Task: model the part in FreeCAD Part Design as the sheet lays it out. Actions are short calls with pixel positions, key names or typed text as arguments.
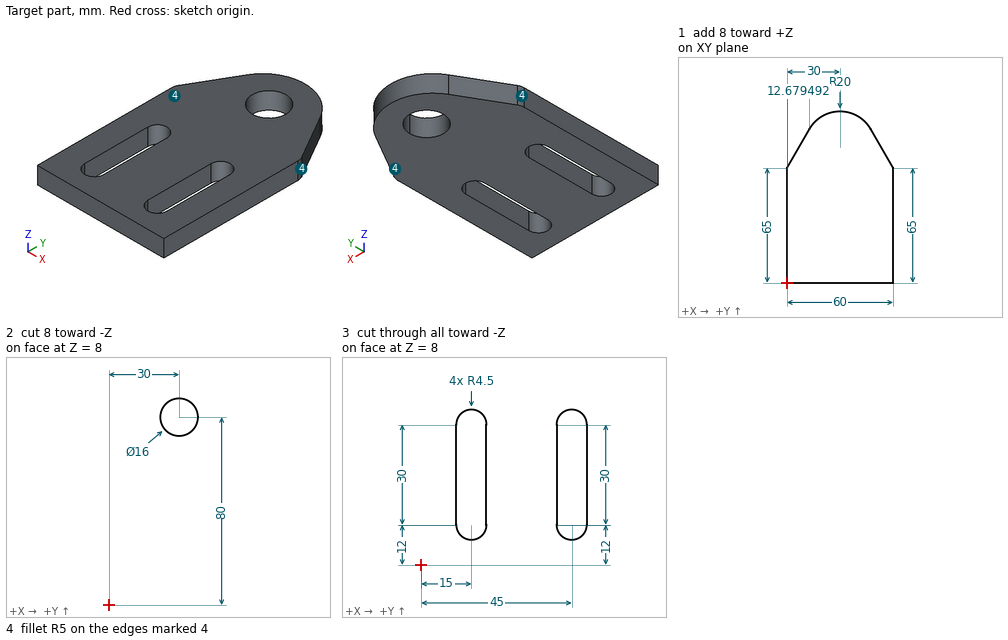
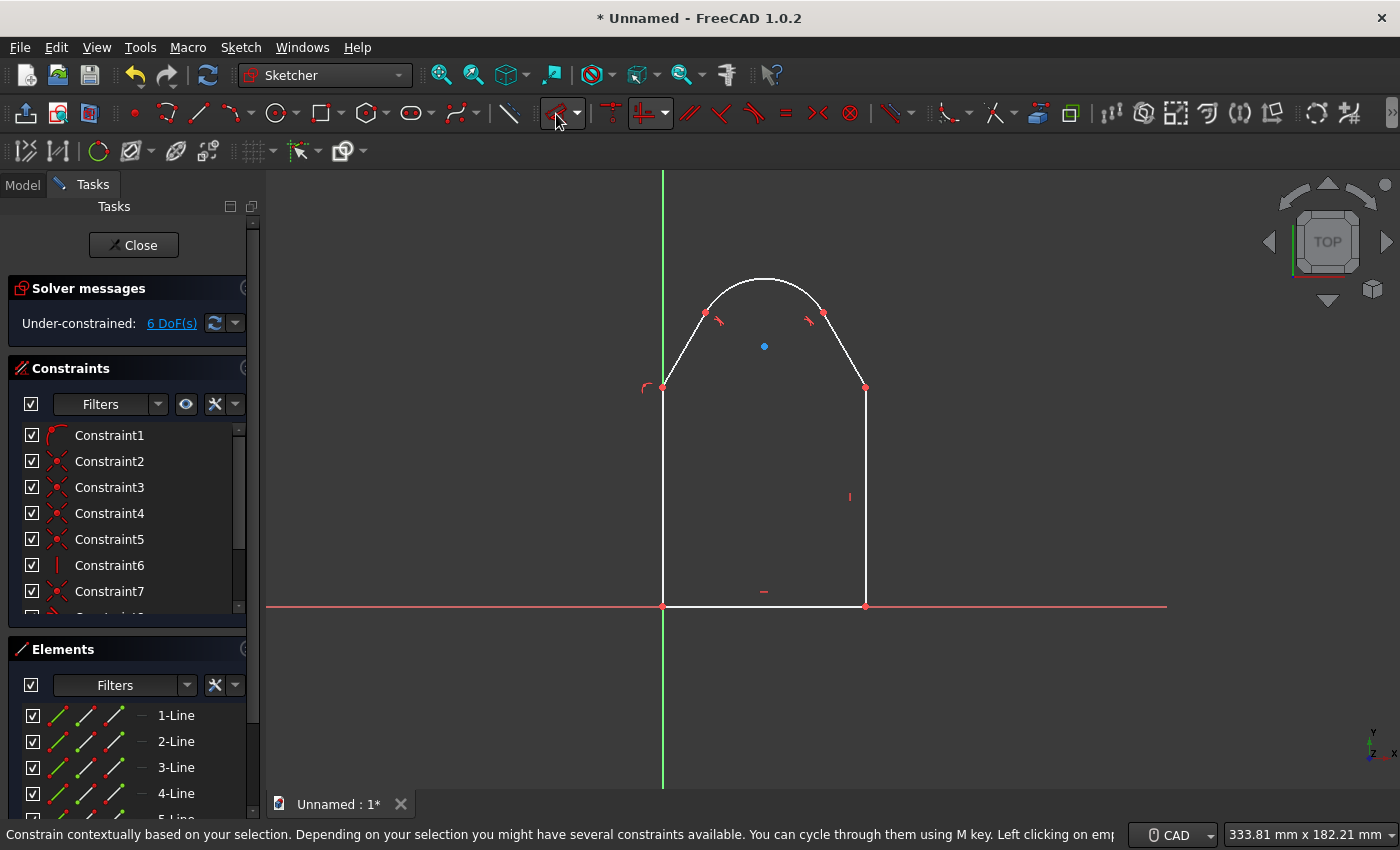
click(792, 285)
click(805, 256)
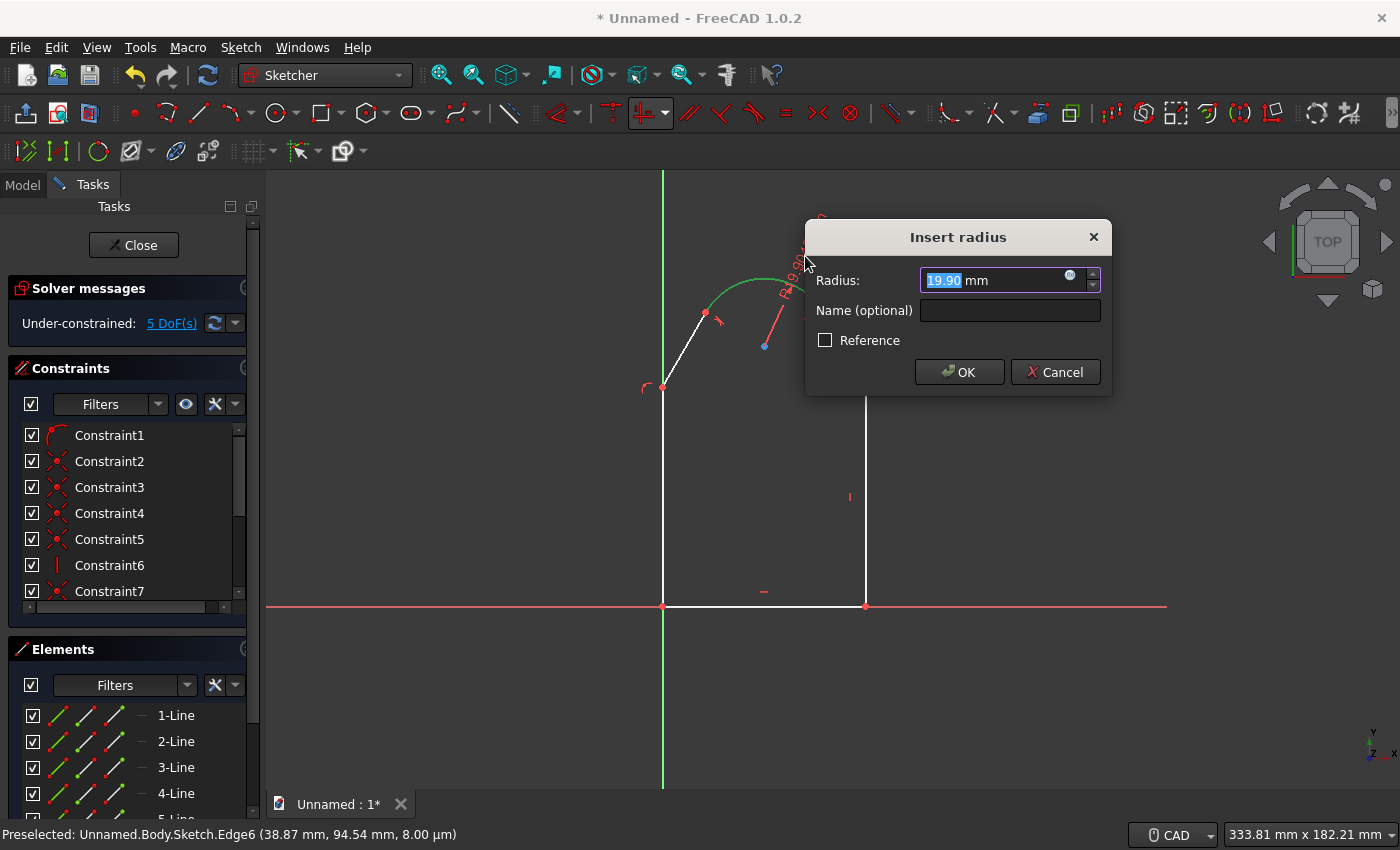
text(20)
key(Return)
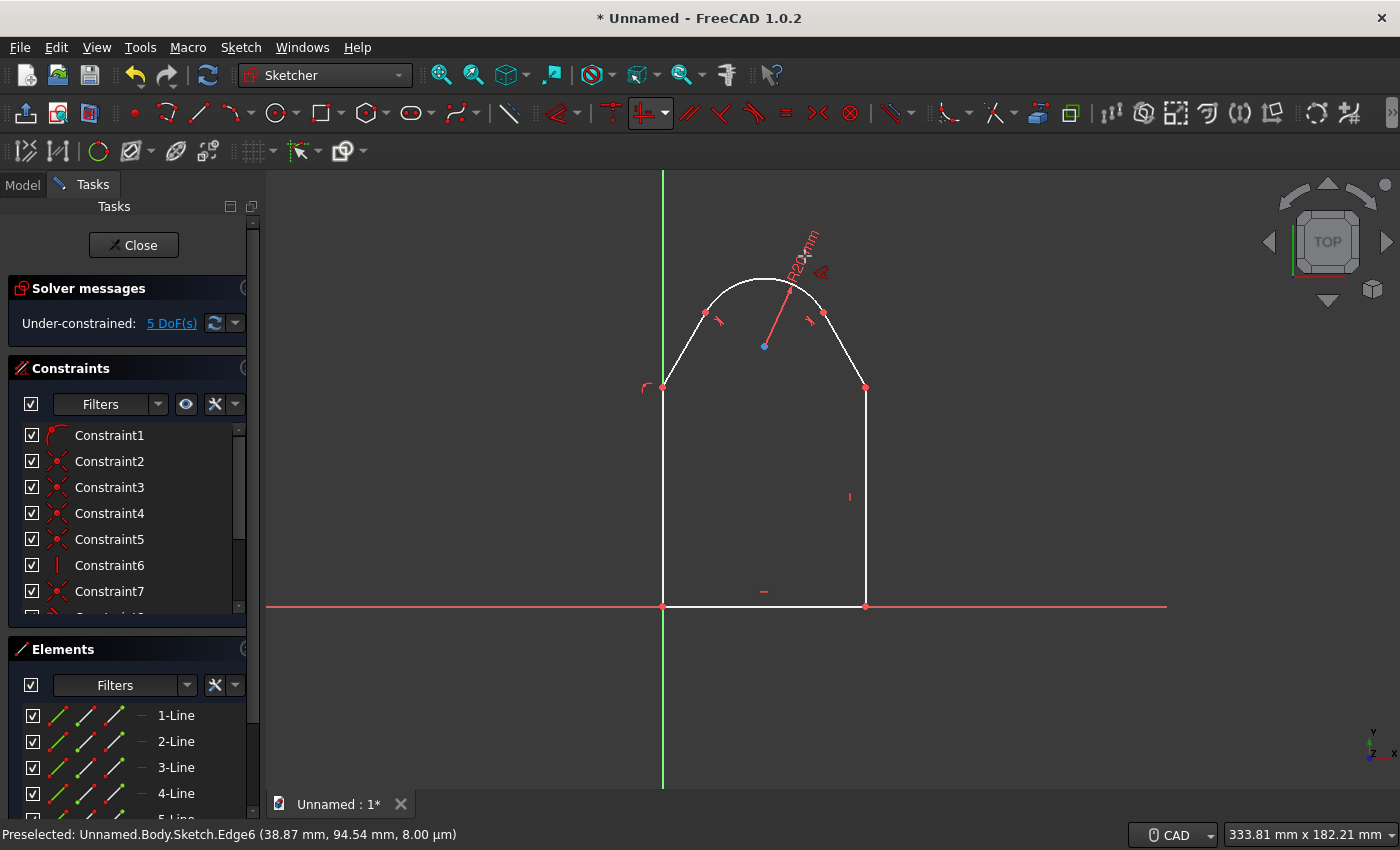
click(663, 453)
click(629, 497)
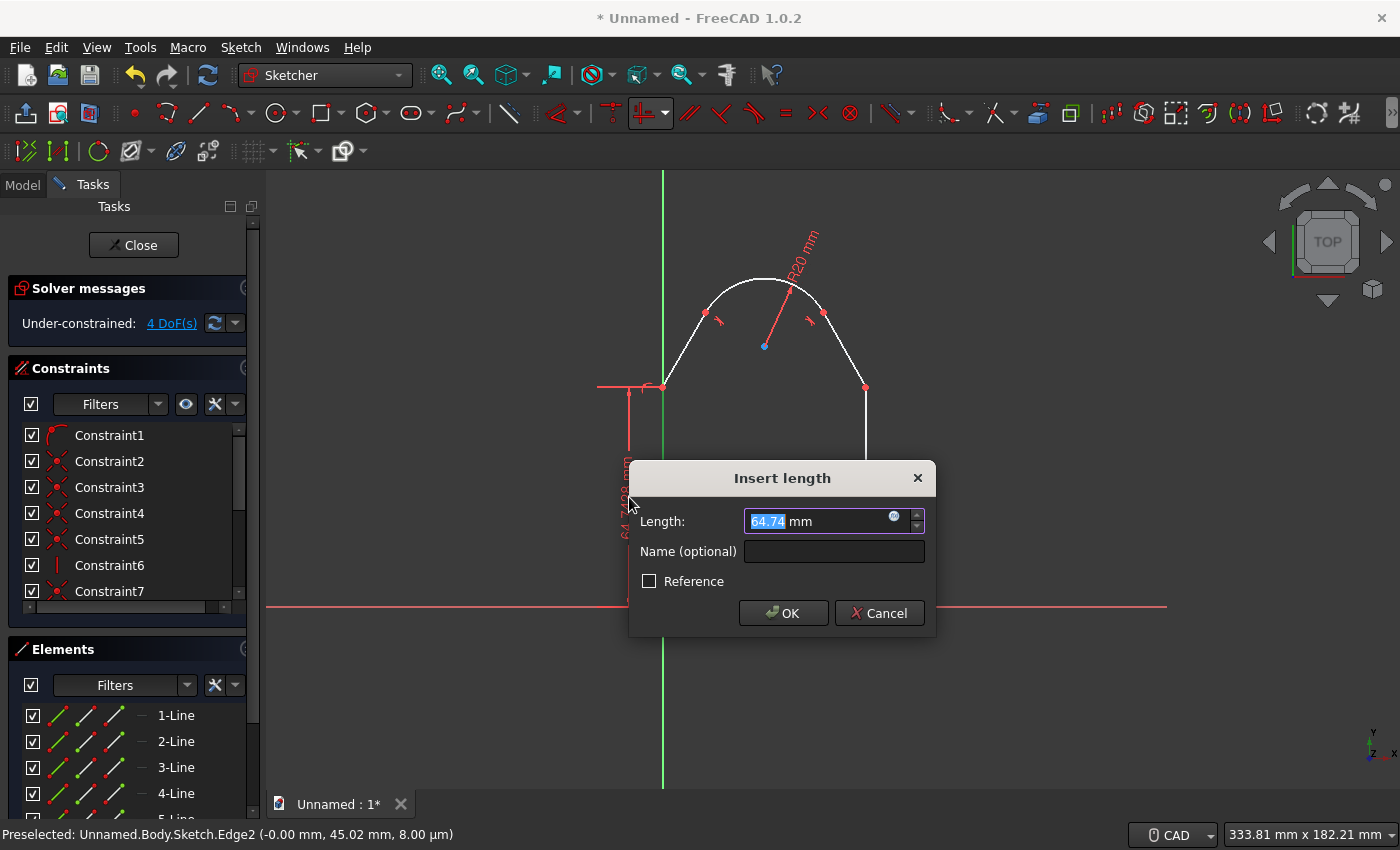
text(65)
key(Return)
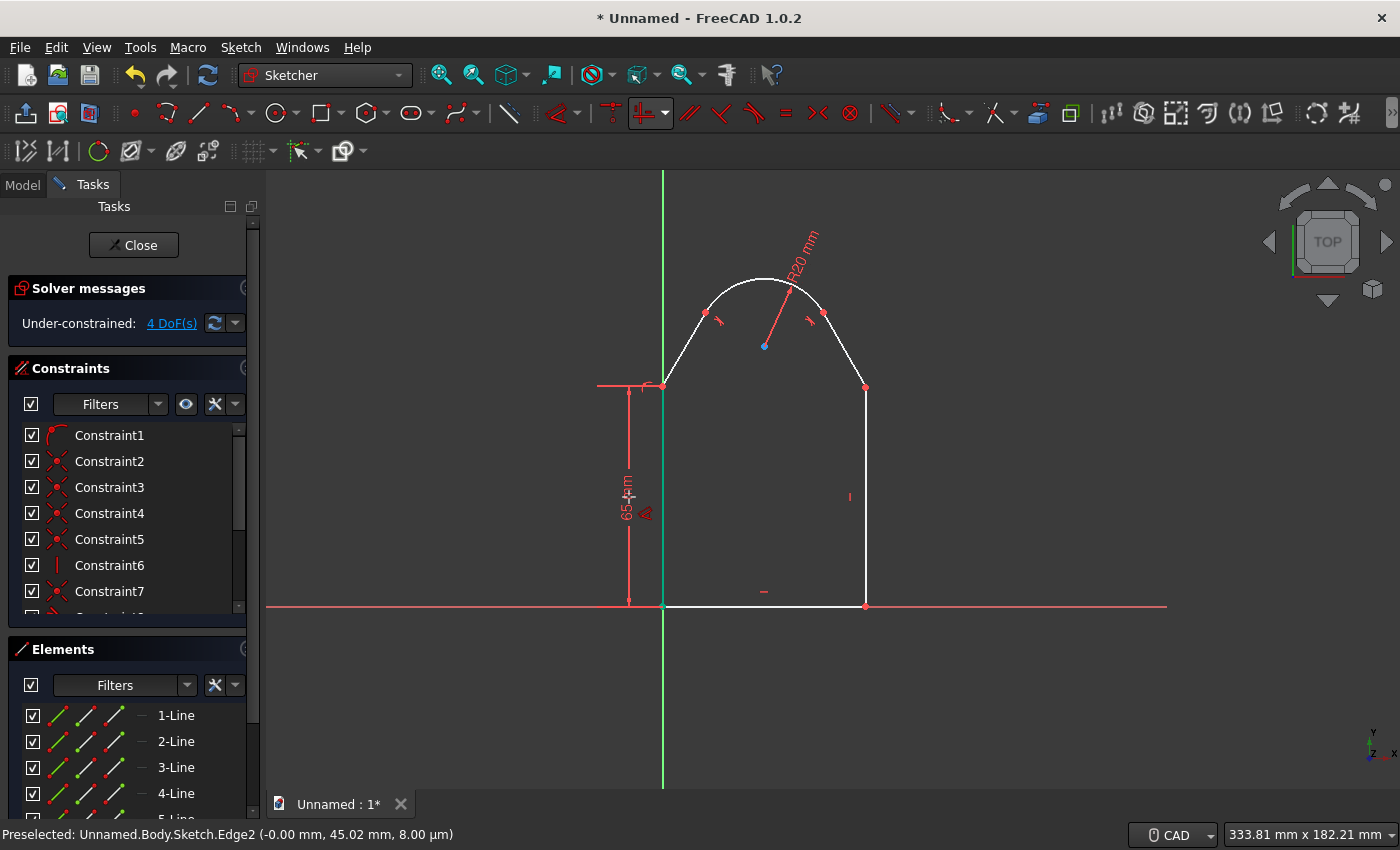
click(724, 607)
click(764, 641)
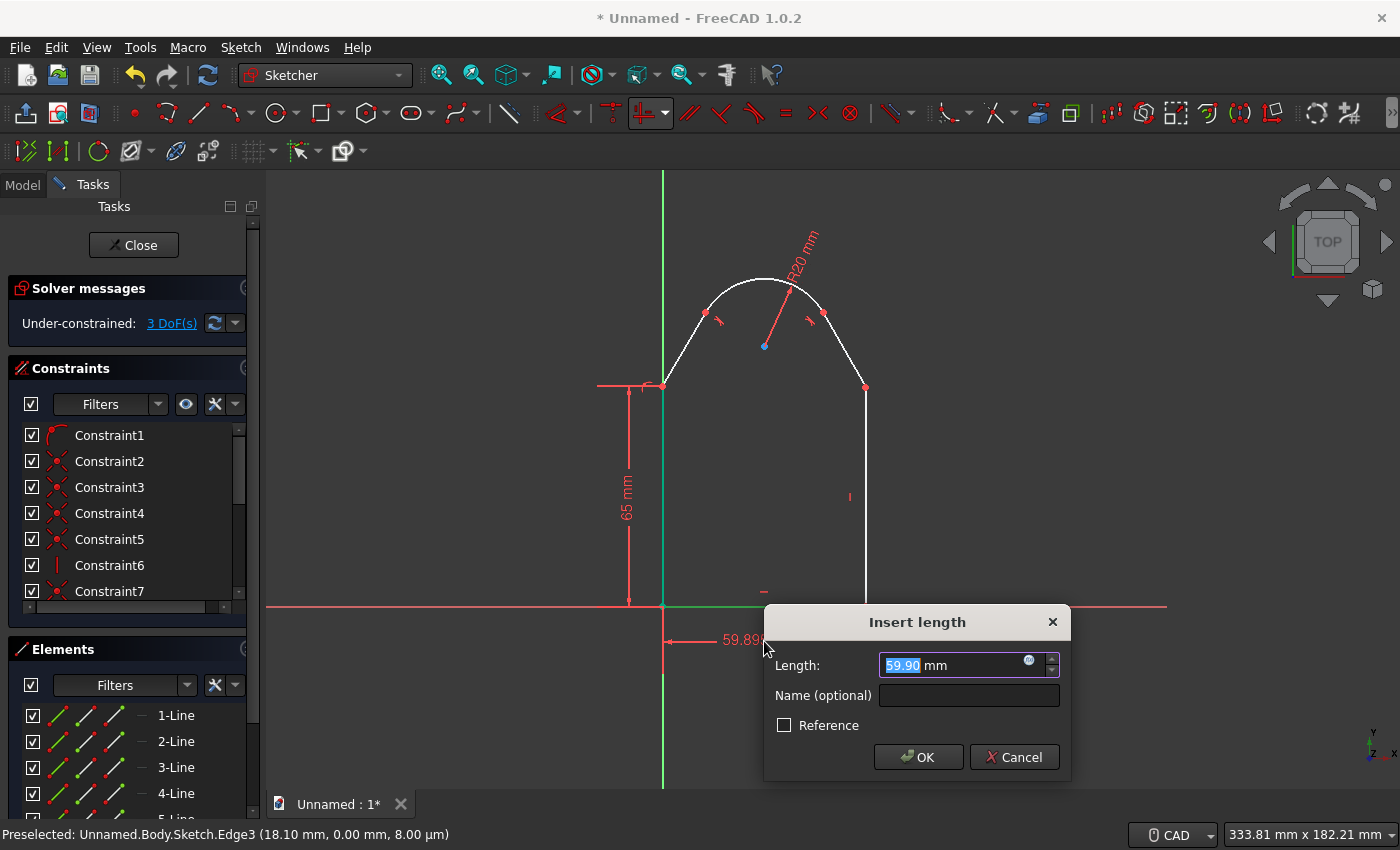
text(60)
key(Return)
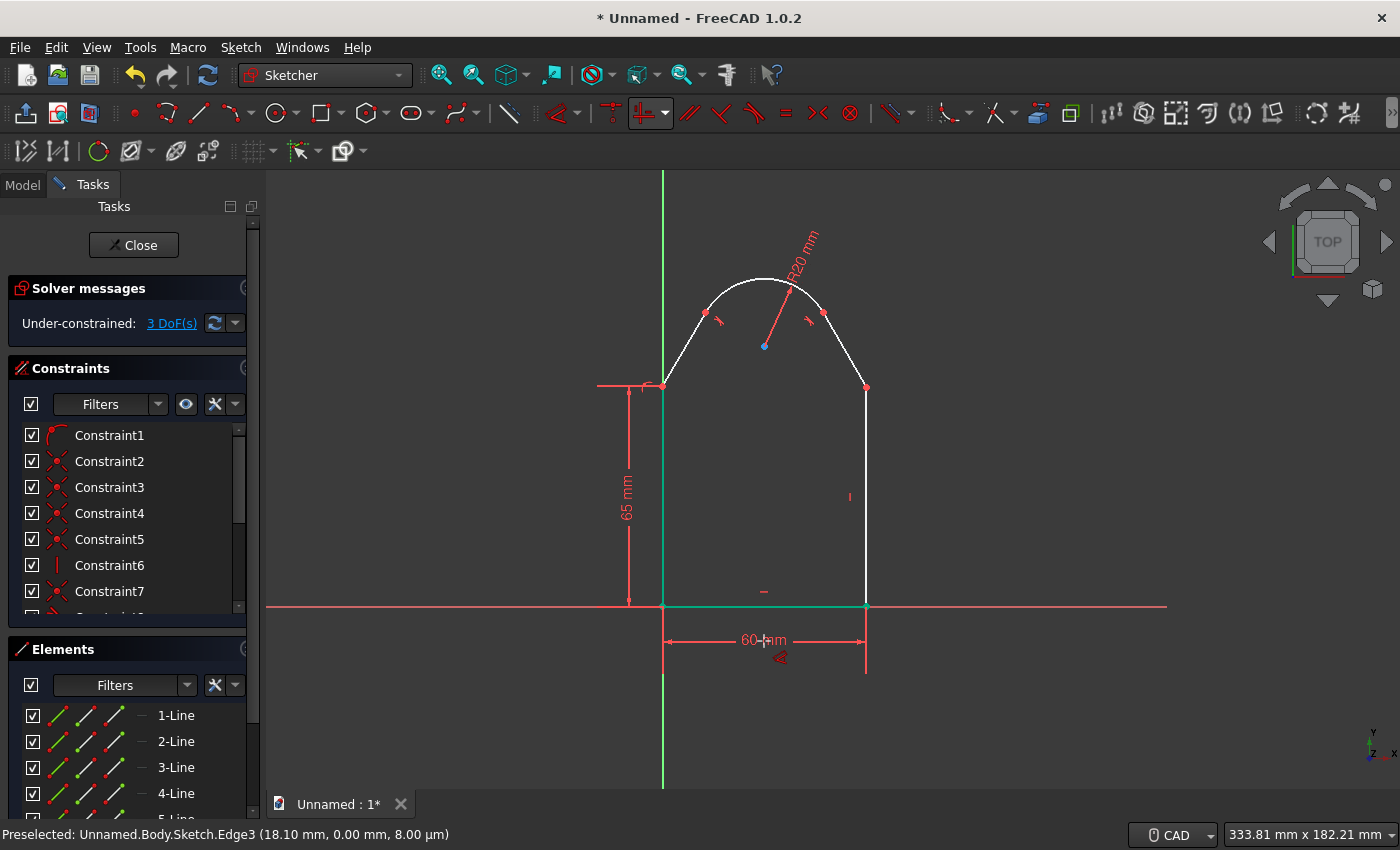
click(866, 541)
click(900, 497)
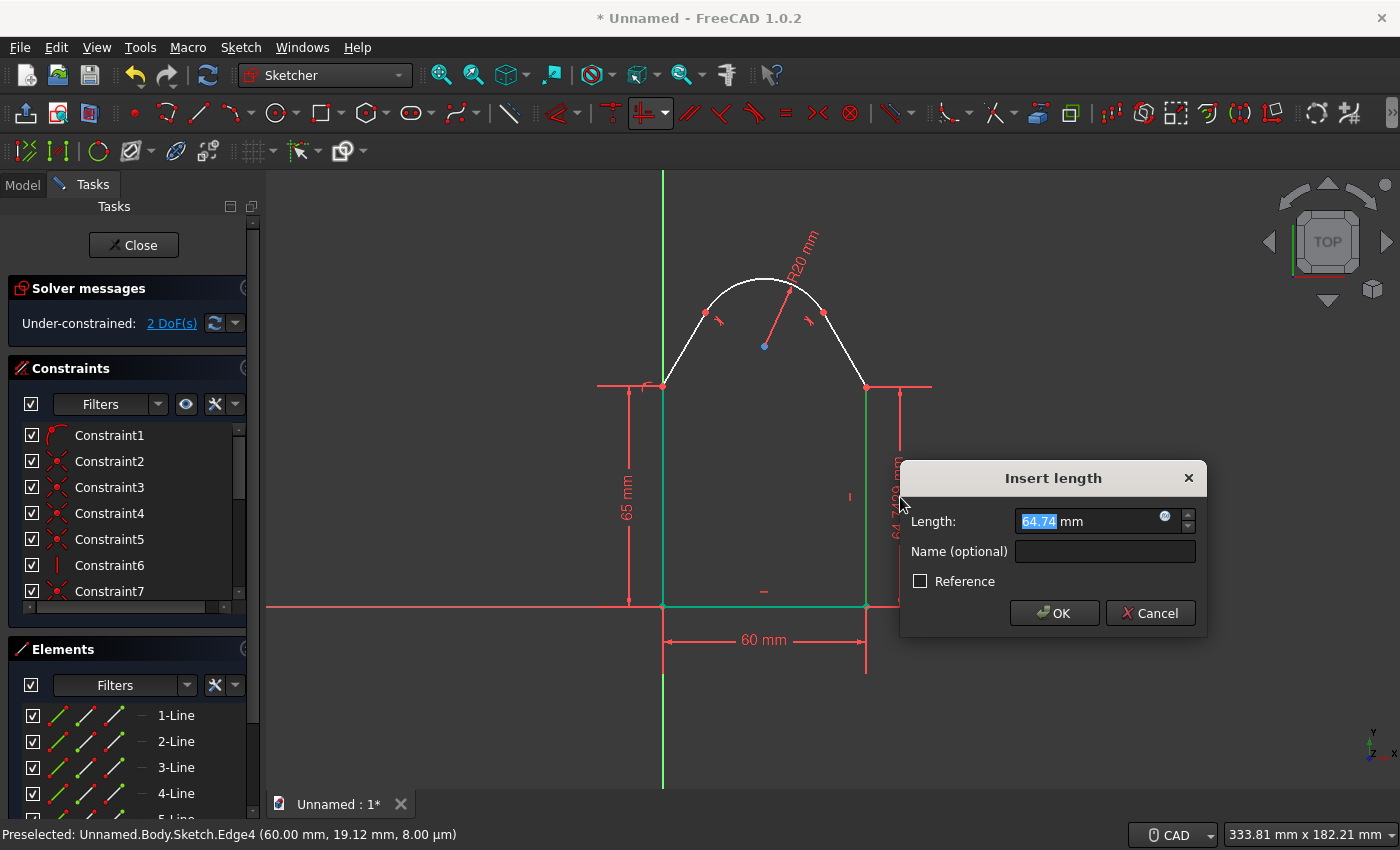
text(65)
key(Return)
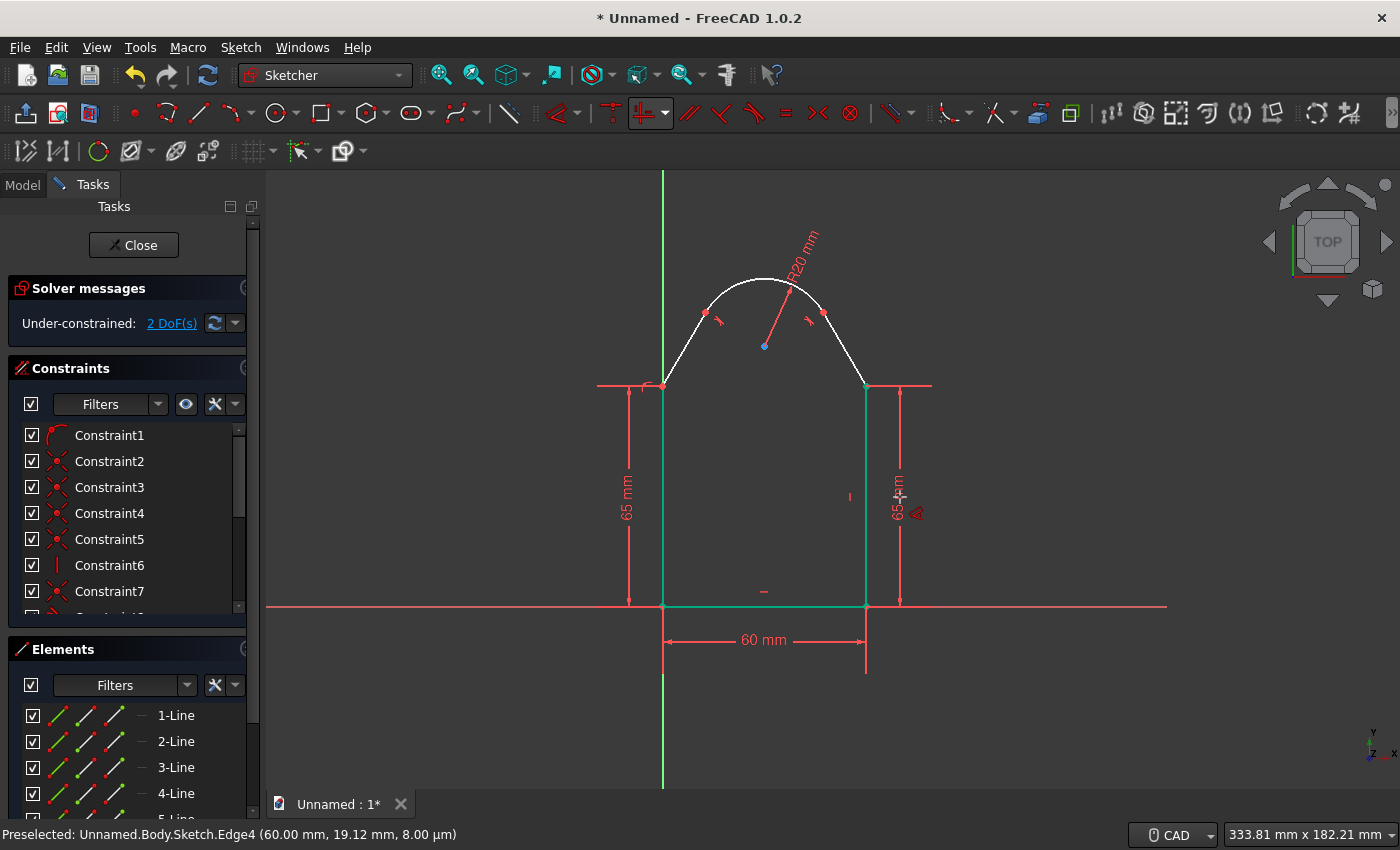
click(765, 347)
click(690, 641)